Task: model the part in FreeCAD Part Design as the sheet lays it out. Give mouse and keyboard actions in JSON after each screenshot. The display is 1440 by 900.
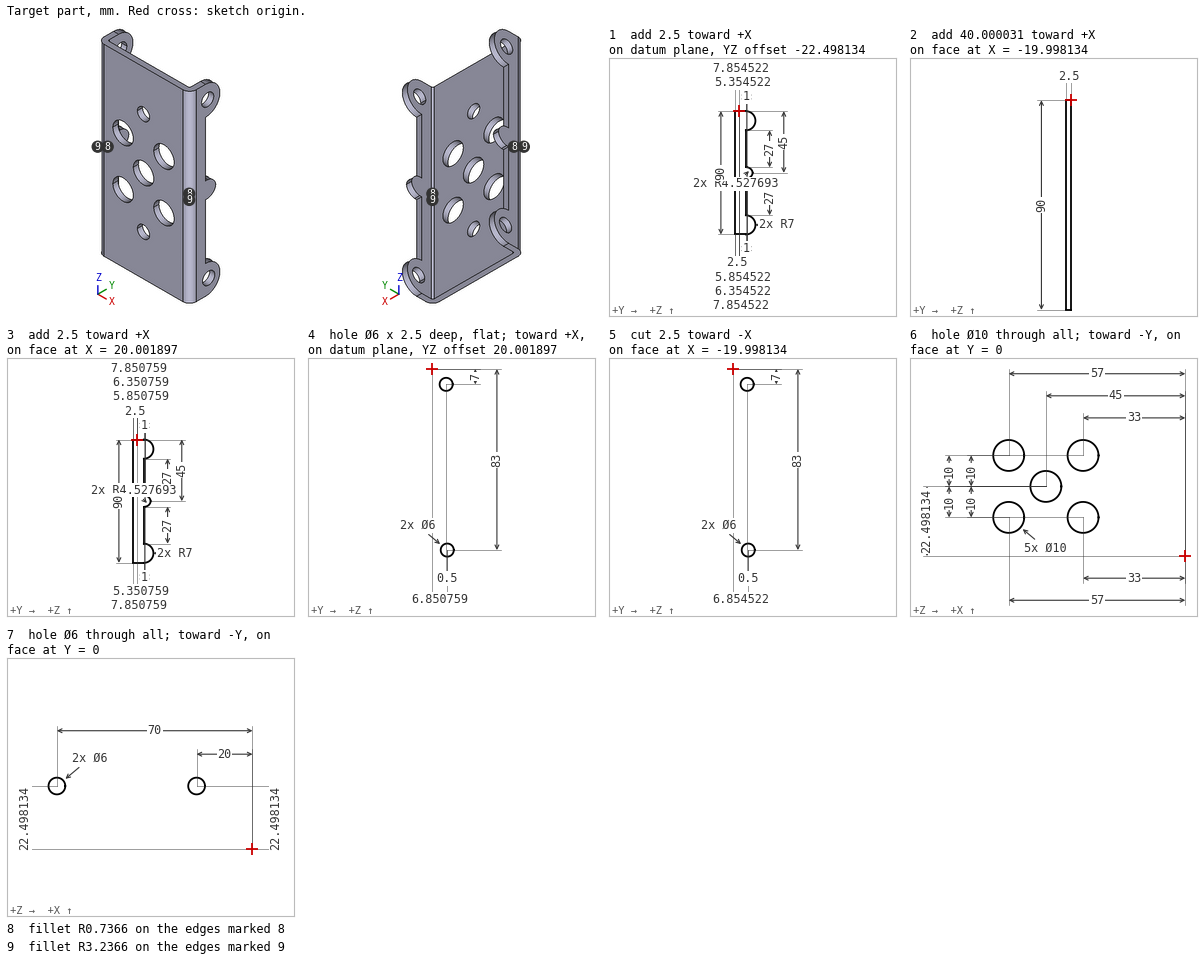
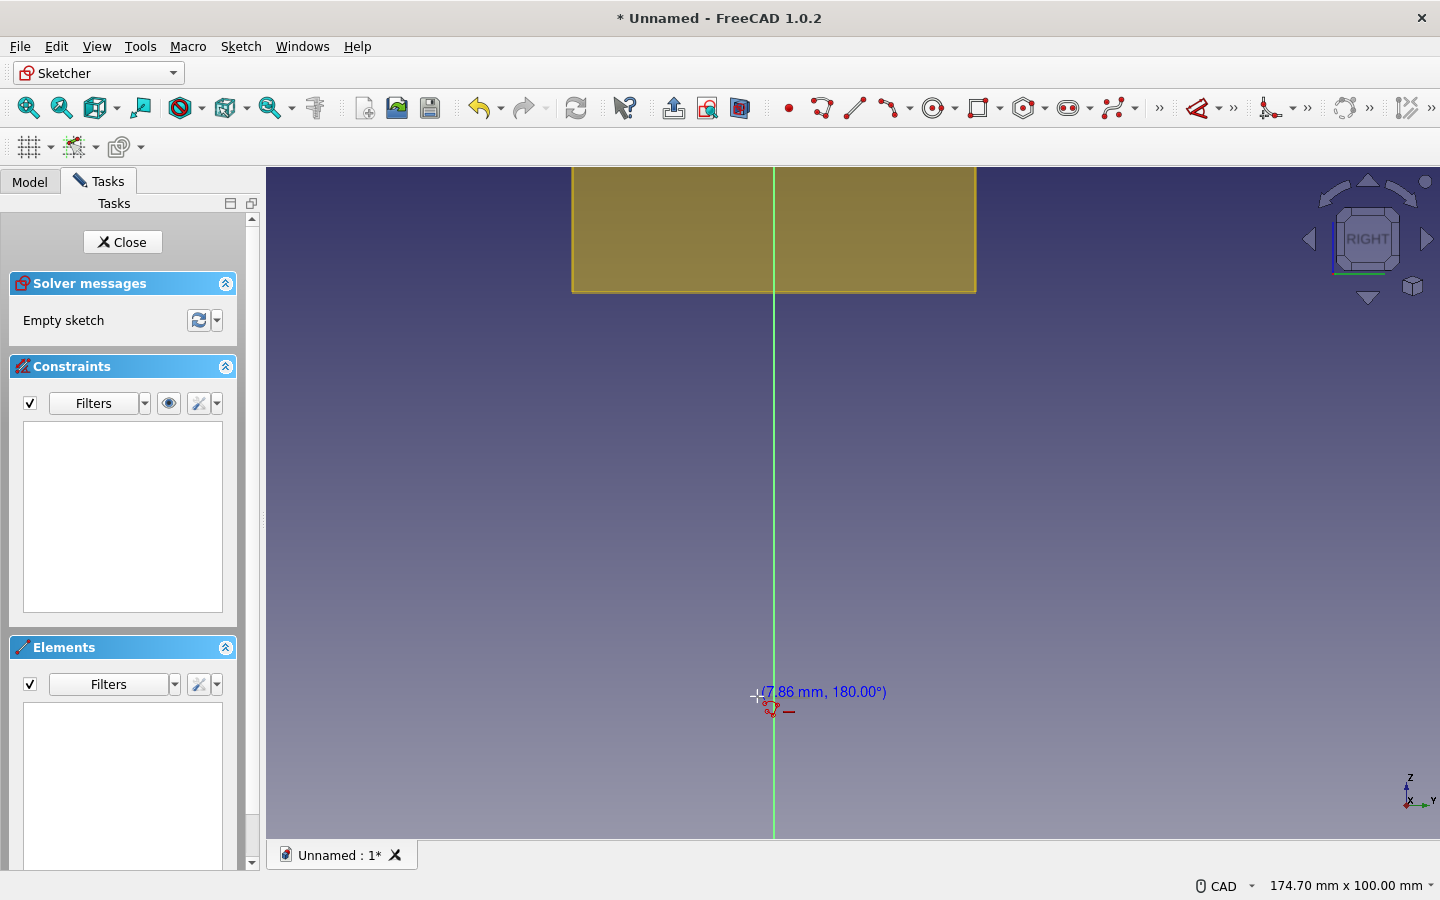
{"action": "left_click", "coordinate": [757, 695]}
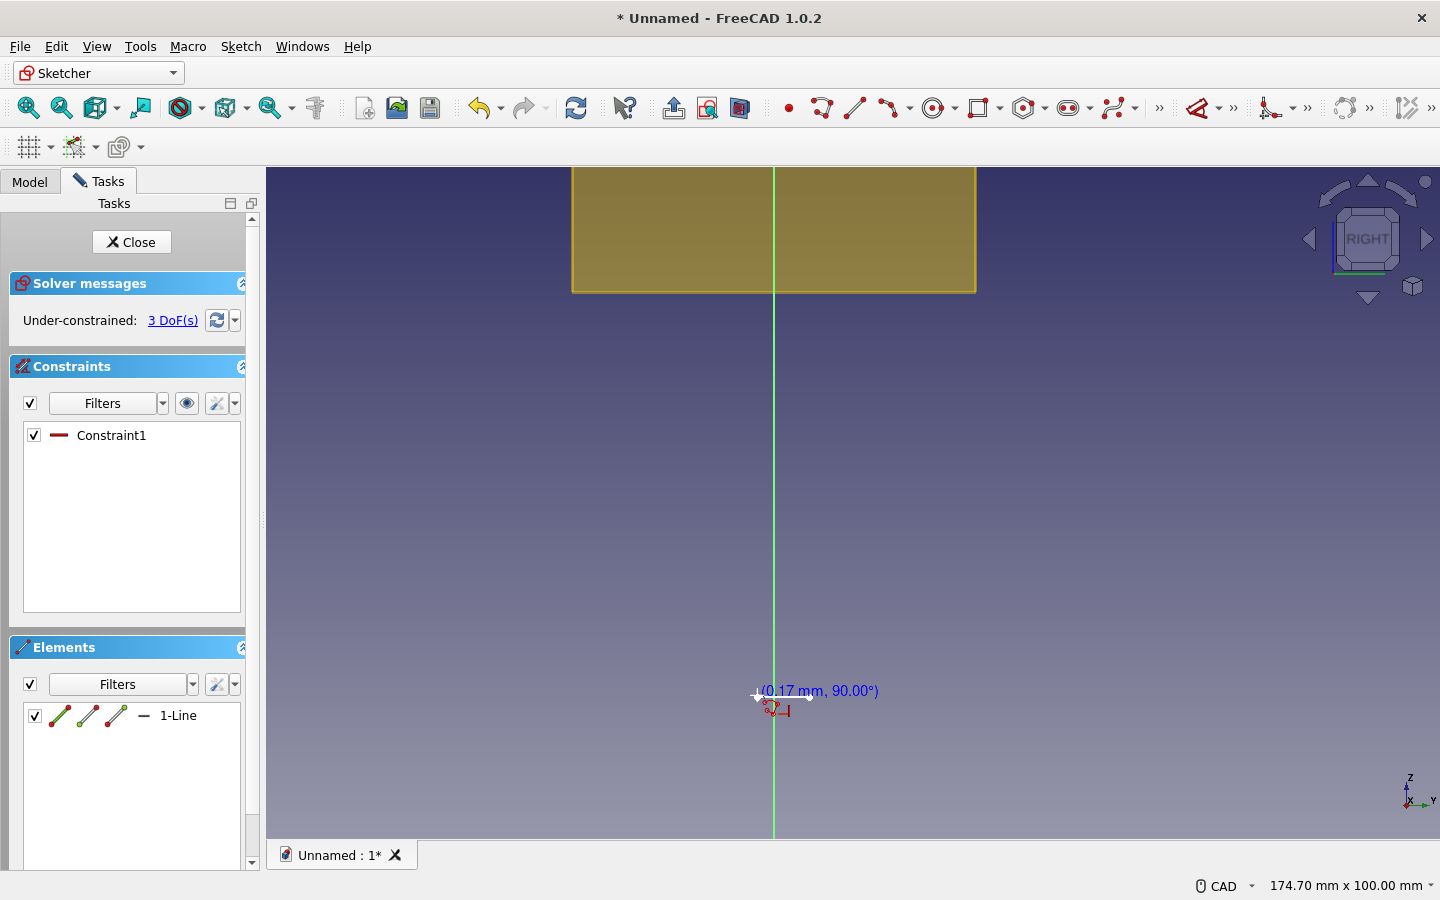
{"action": "scroll", "coordinate": [739, 727], "scroll_direction": "down", "scroll_amount": 2}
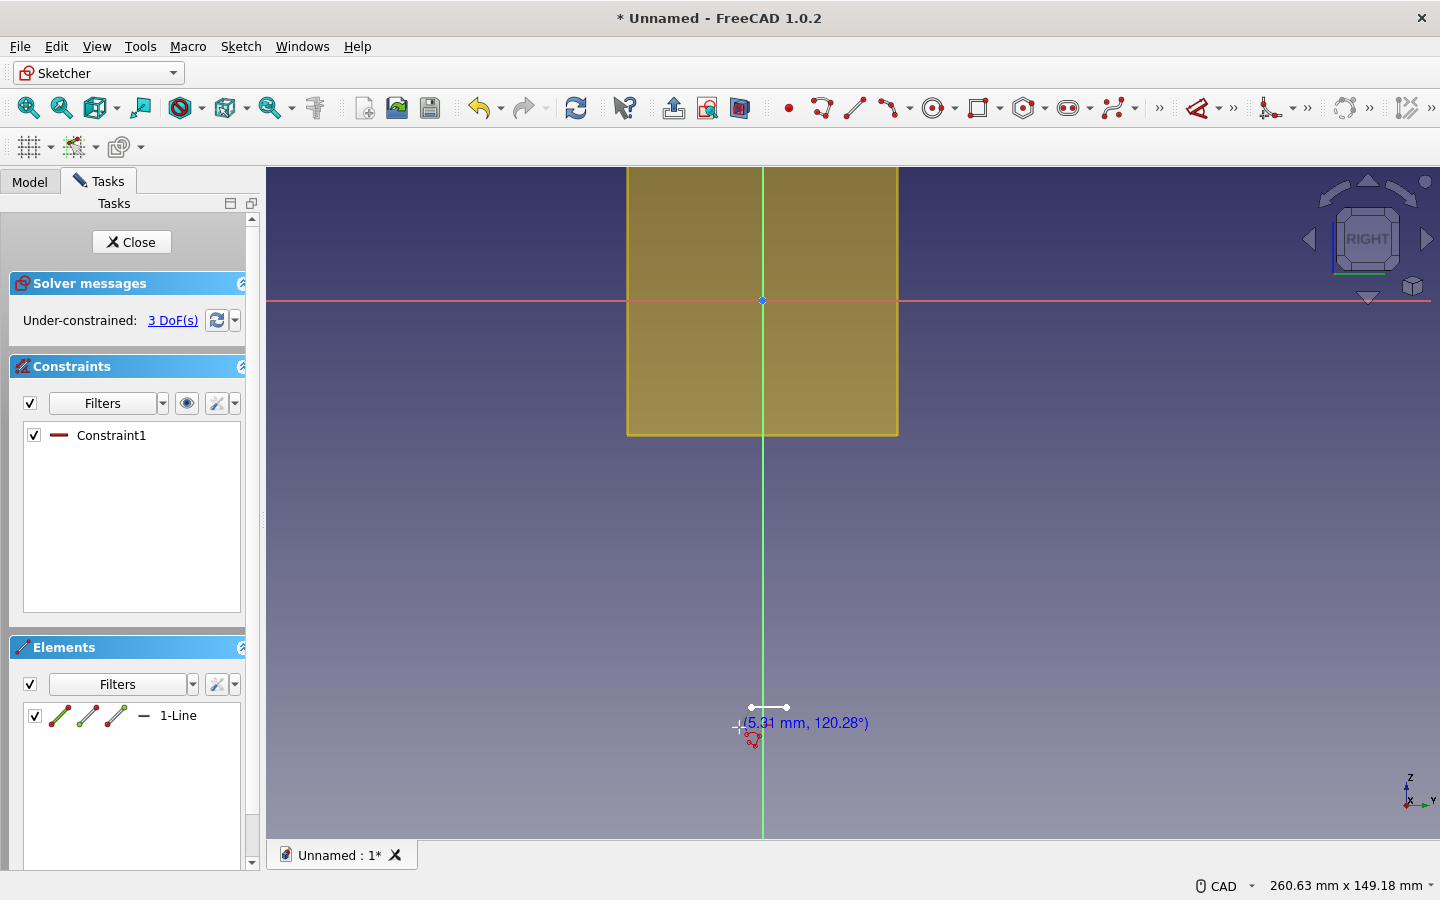
{"action": "scroll", "coordinate": [751, 301], "scroll_direction": "up", "scroll_amount": 2}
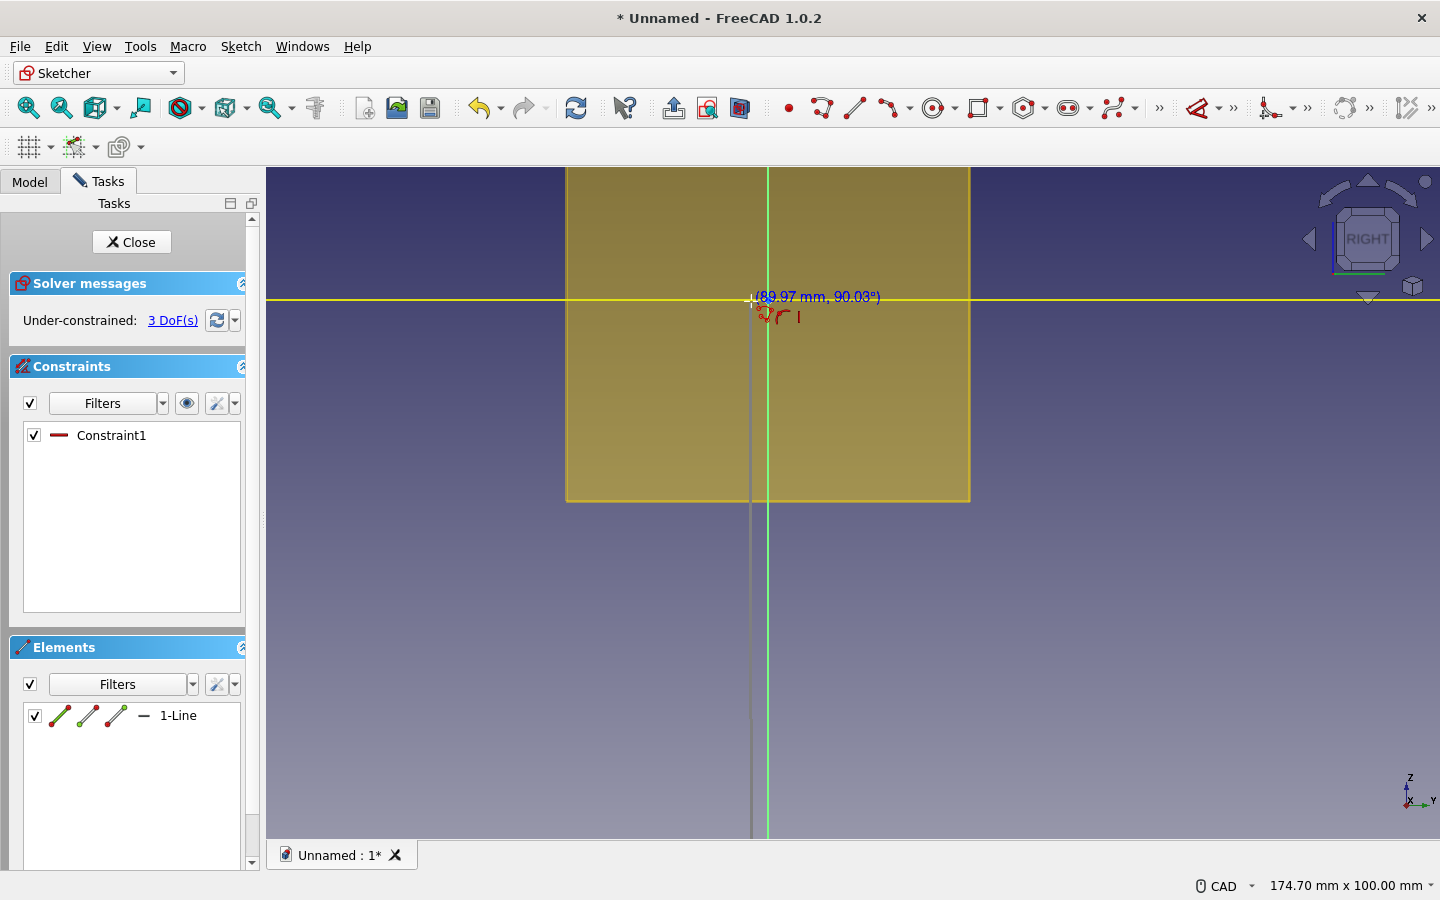
{"action": "left_click", "coordinate": [751, 300]}
{"action": "left_click", "coordinate": [804, 309]}
{"action": "right_click", "coordinate": [804, 309]}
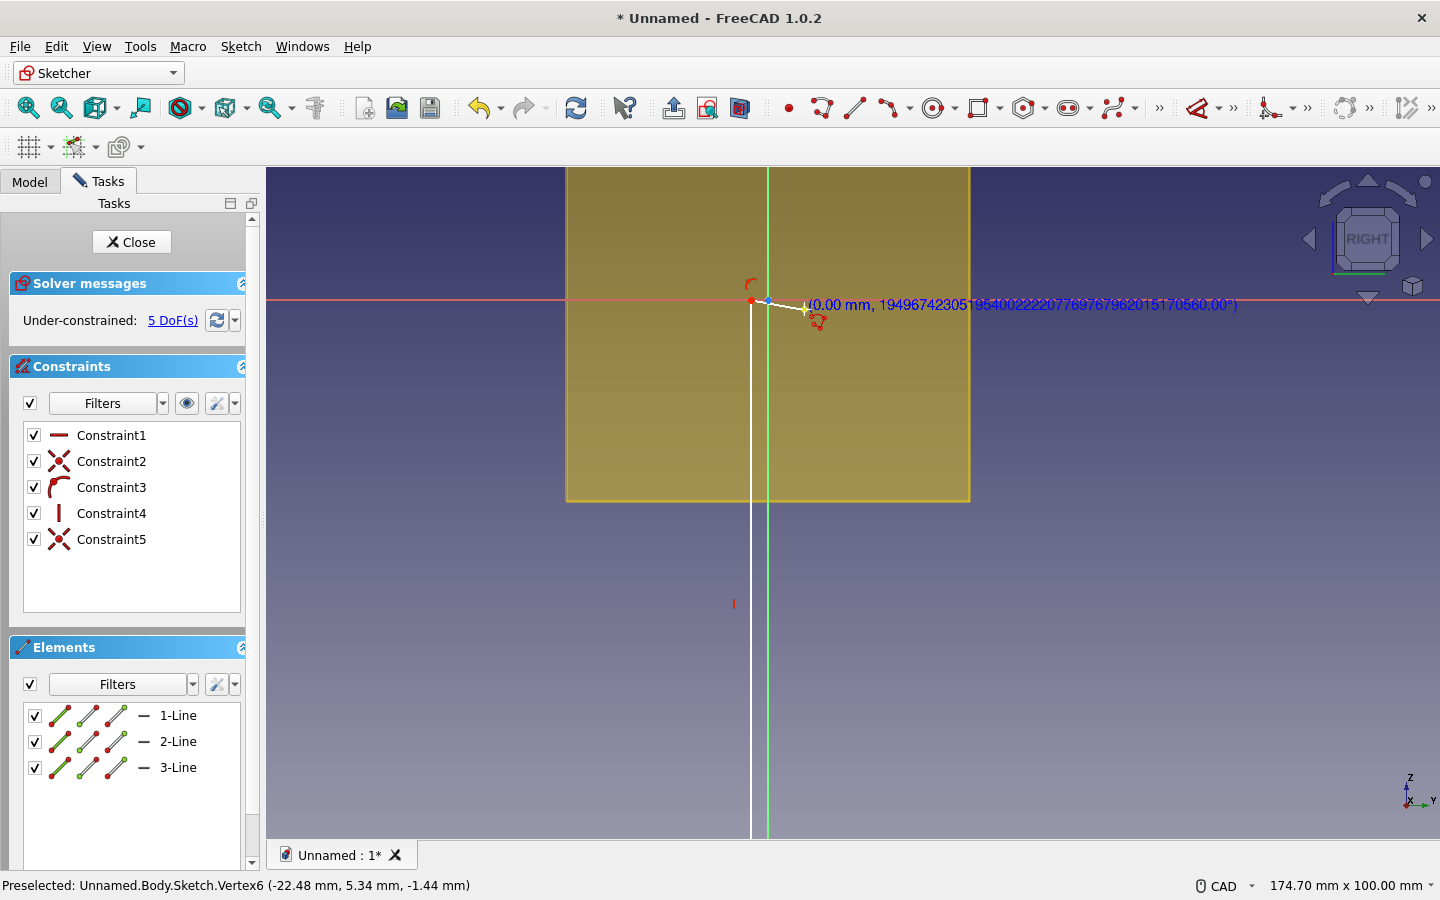
{"action": "left_click", "coordinate": [804, 394]}
{"action": "left_click", "coordinate": [804, 576]}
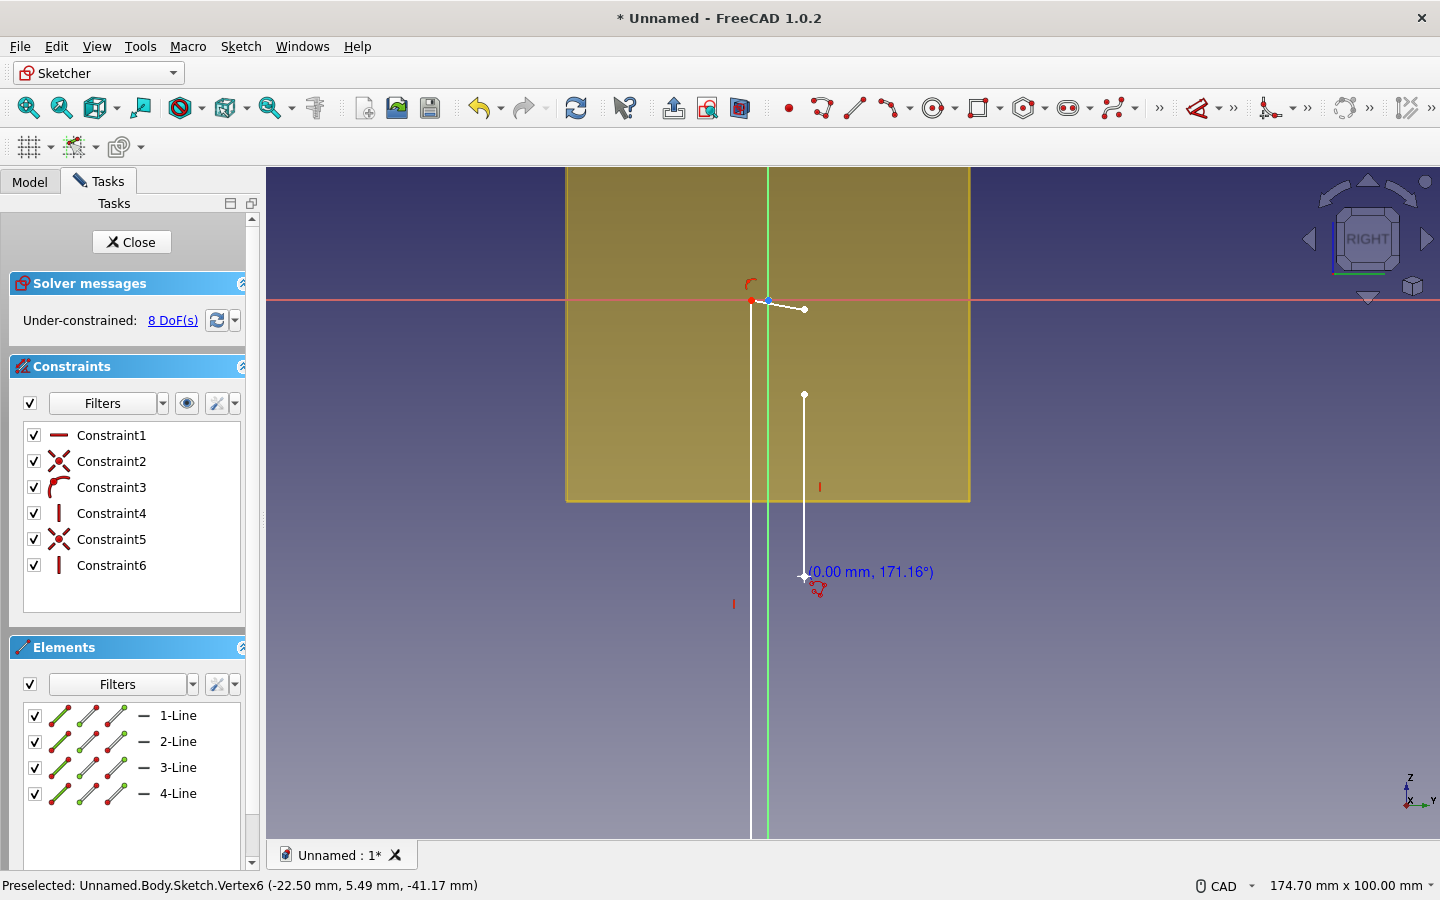
{"action": "scroll", "coordinate": [811, 576], "scroll_direction": "up", "scroll_amount": 5}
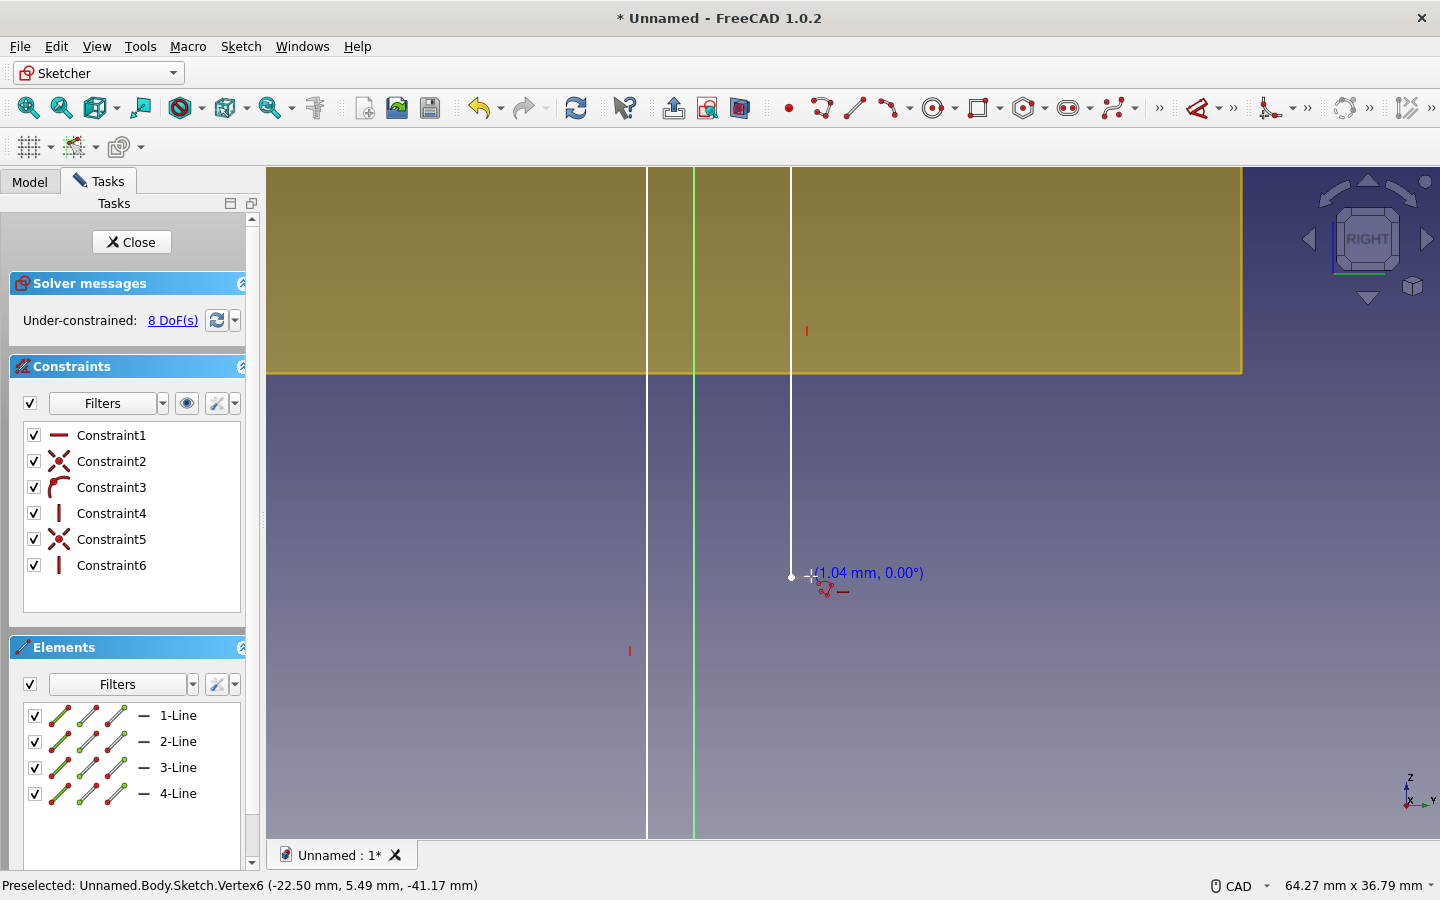
{"action": "left_click", "coordinate": [810, 575]}
{"action": "right_click", "coordinate": [810, 575]}